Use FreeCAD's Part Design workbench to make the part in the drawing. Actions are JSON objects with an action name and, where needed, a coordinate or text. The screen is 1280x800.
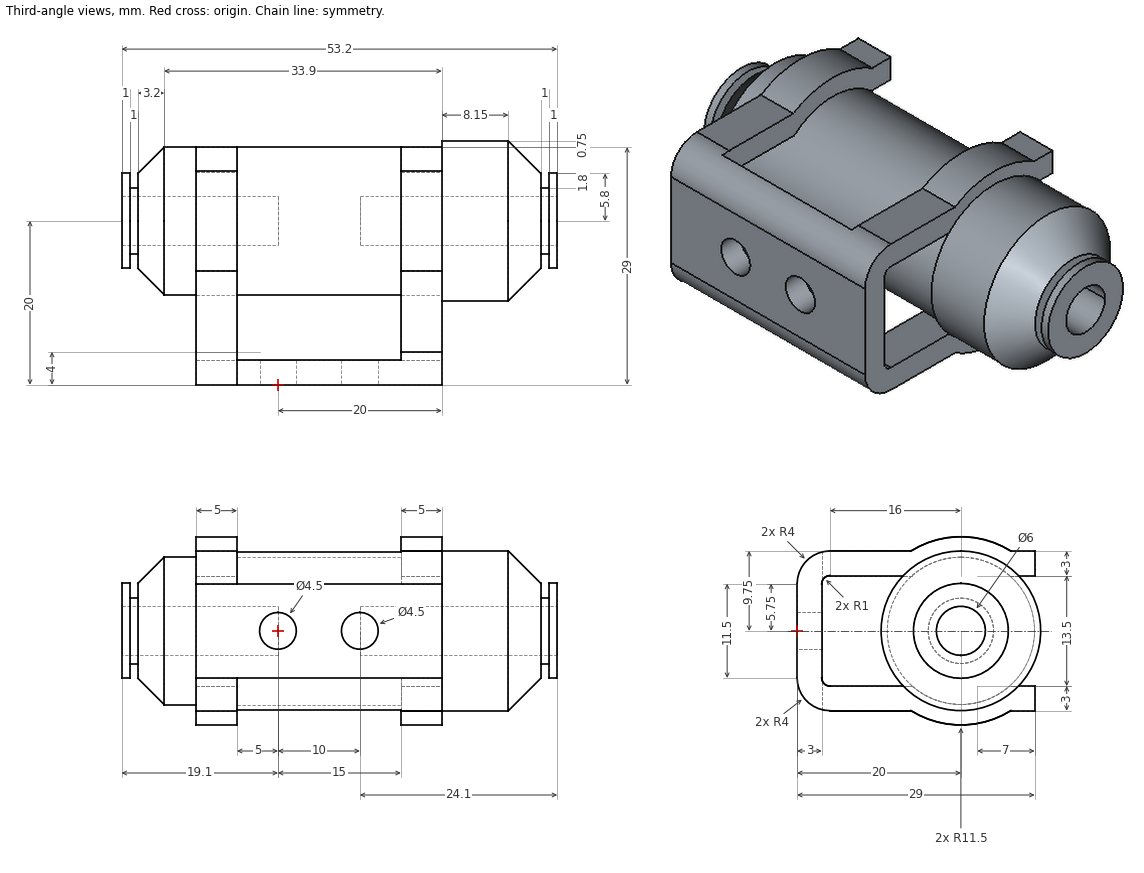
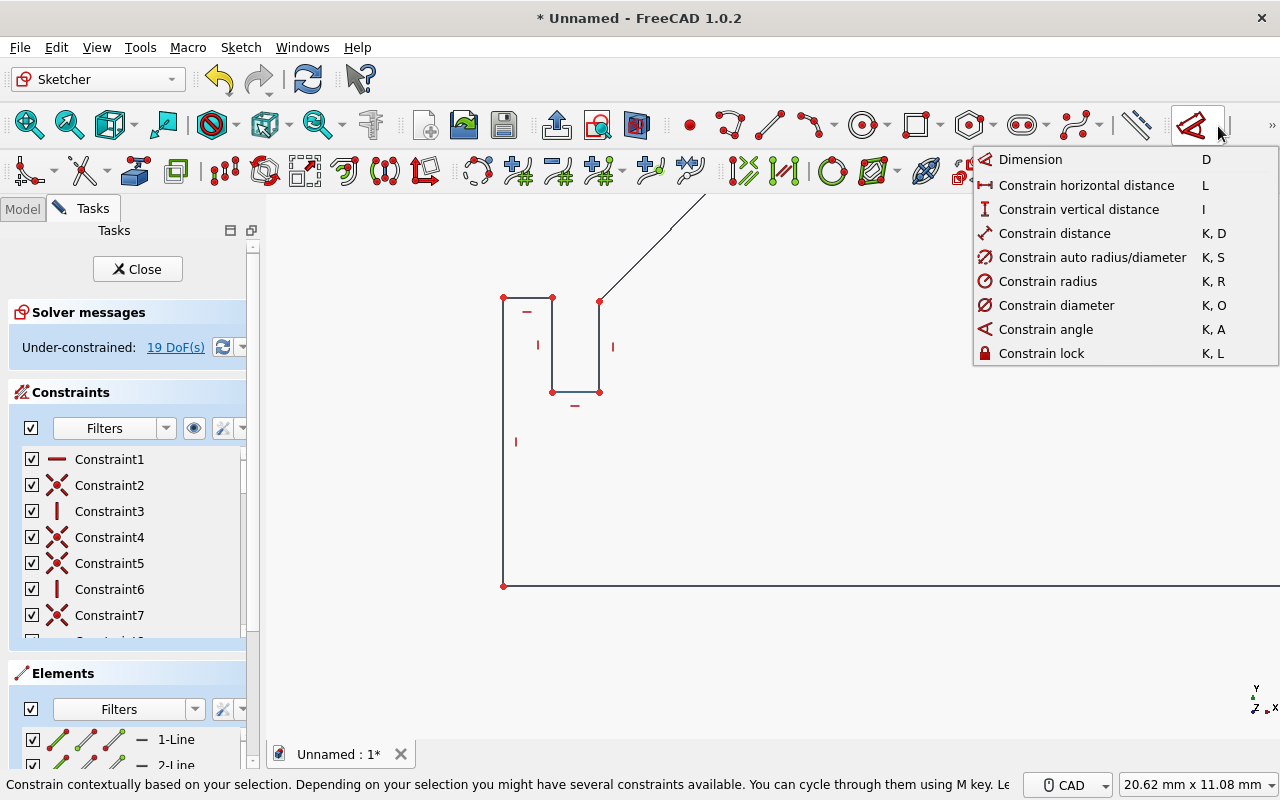
{"action": "left_click", "coordinate": [1126, 185]}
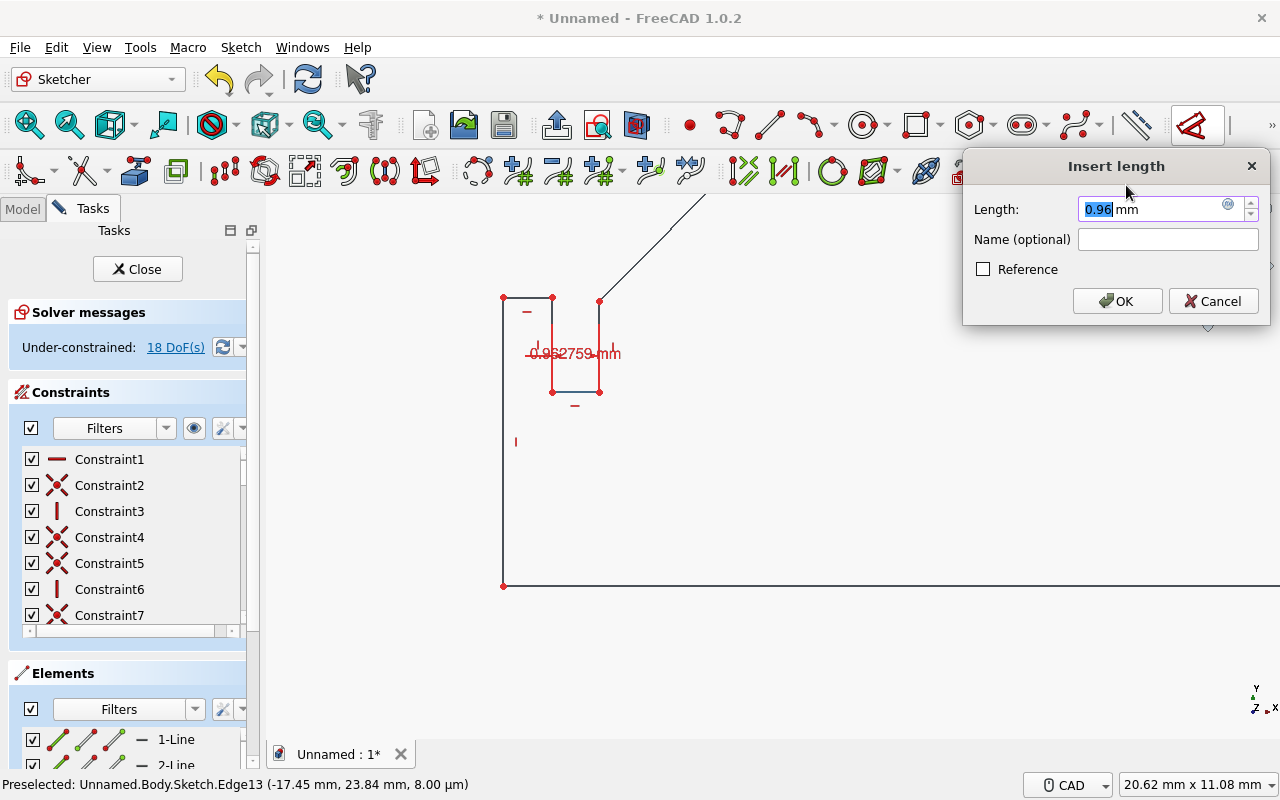
{"action": "type", "text": "1"}
{"action": "key", "text": "Return"}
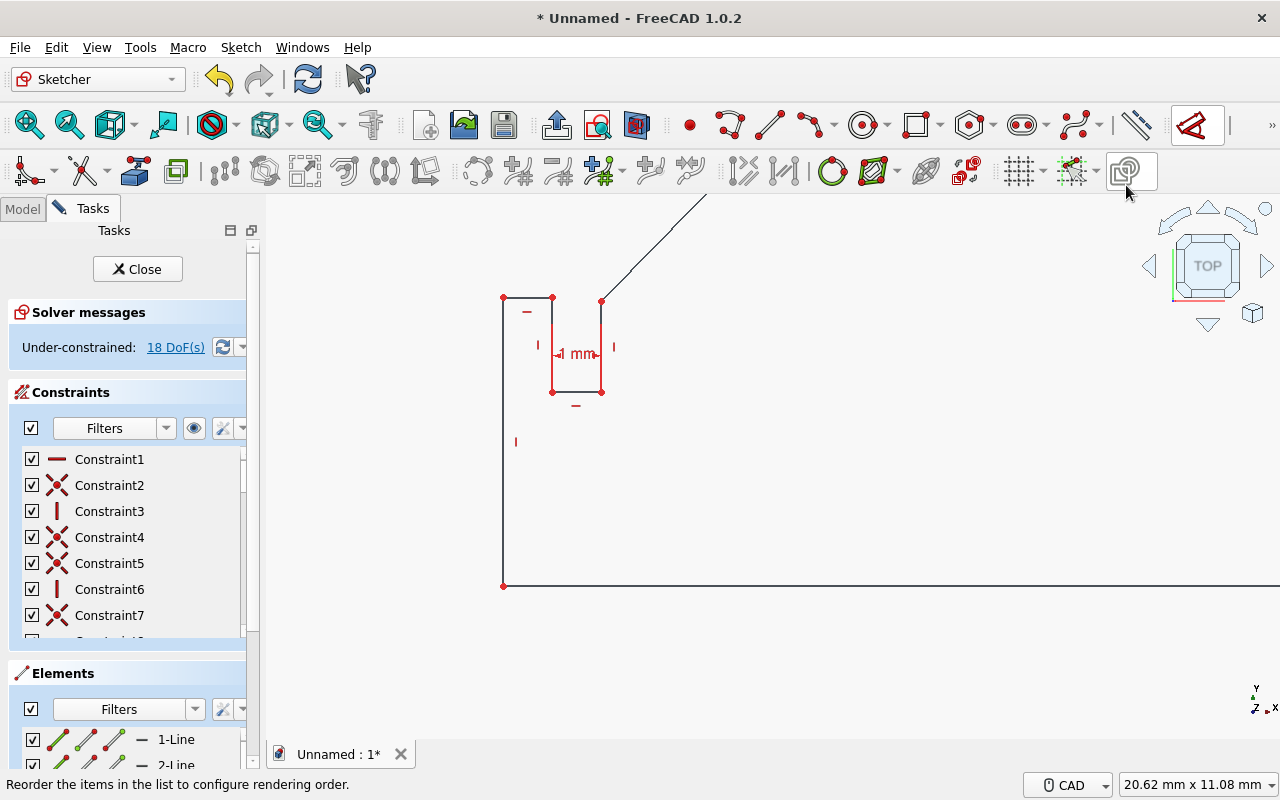
{"action": "left_click", "coordinate": [537, 298]}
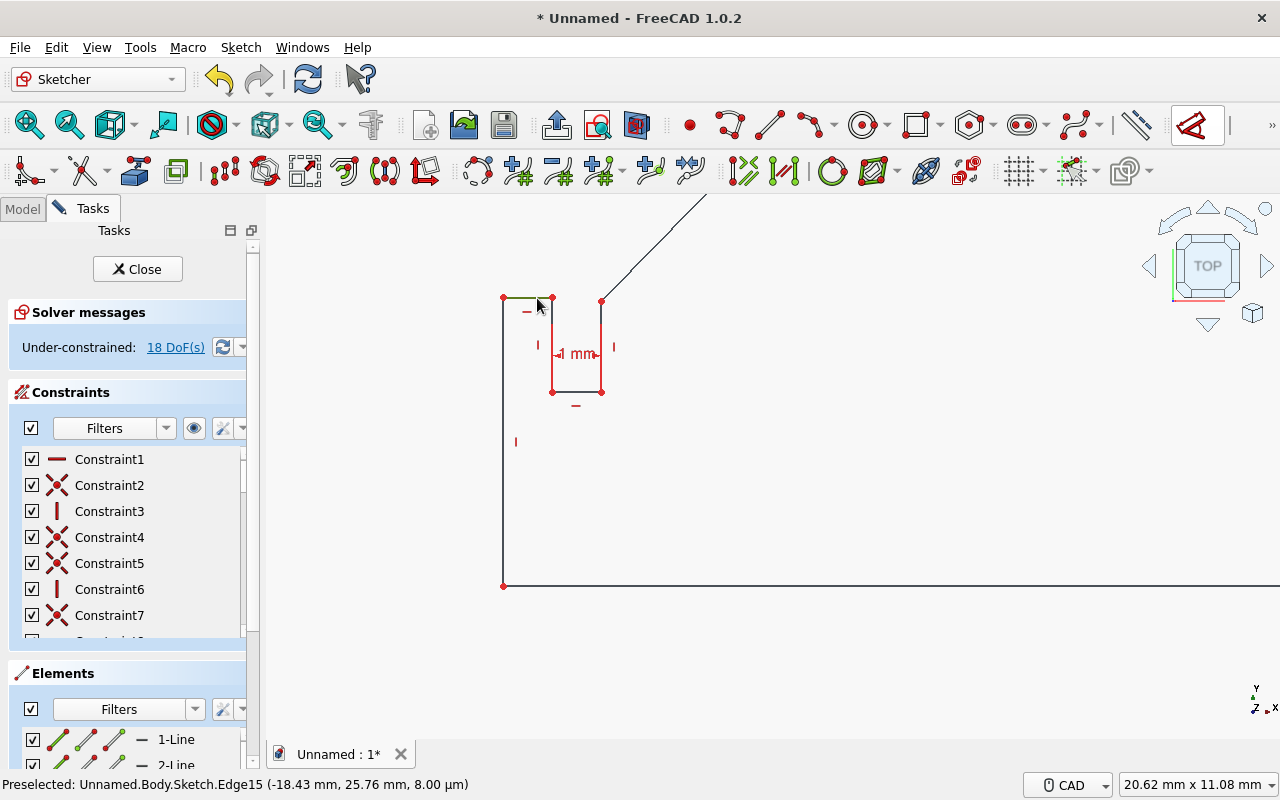
{"action": "key", "text": "l"}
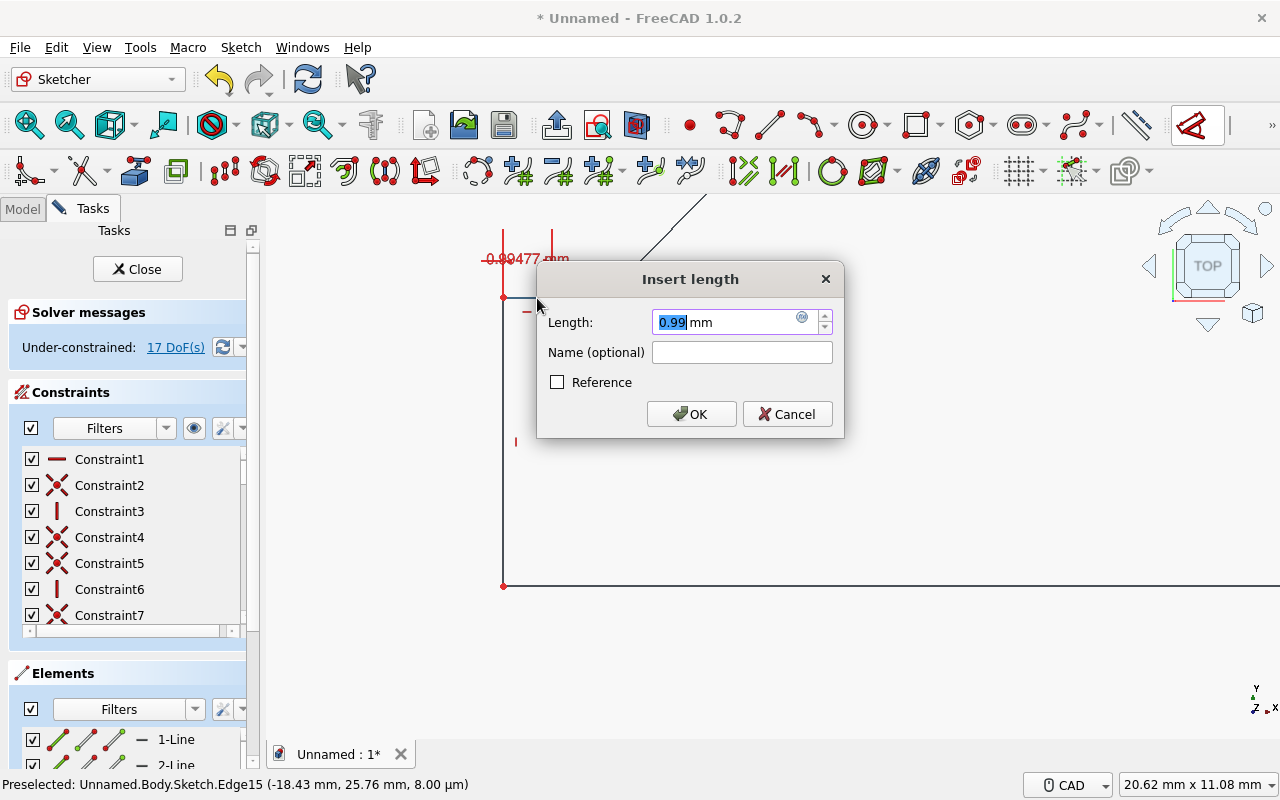
{"action": "type", "text": "1"}
{"action": "key", "text": "Return"}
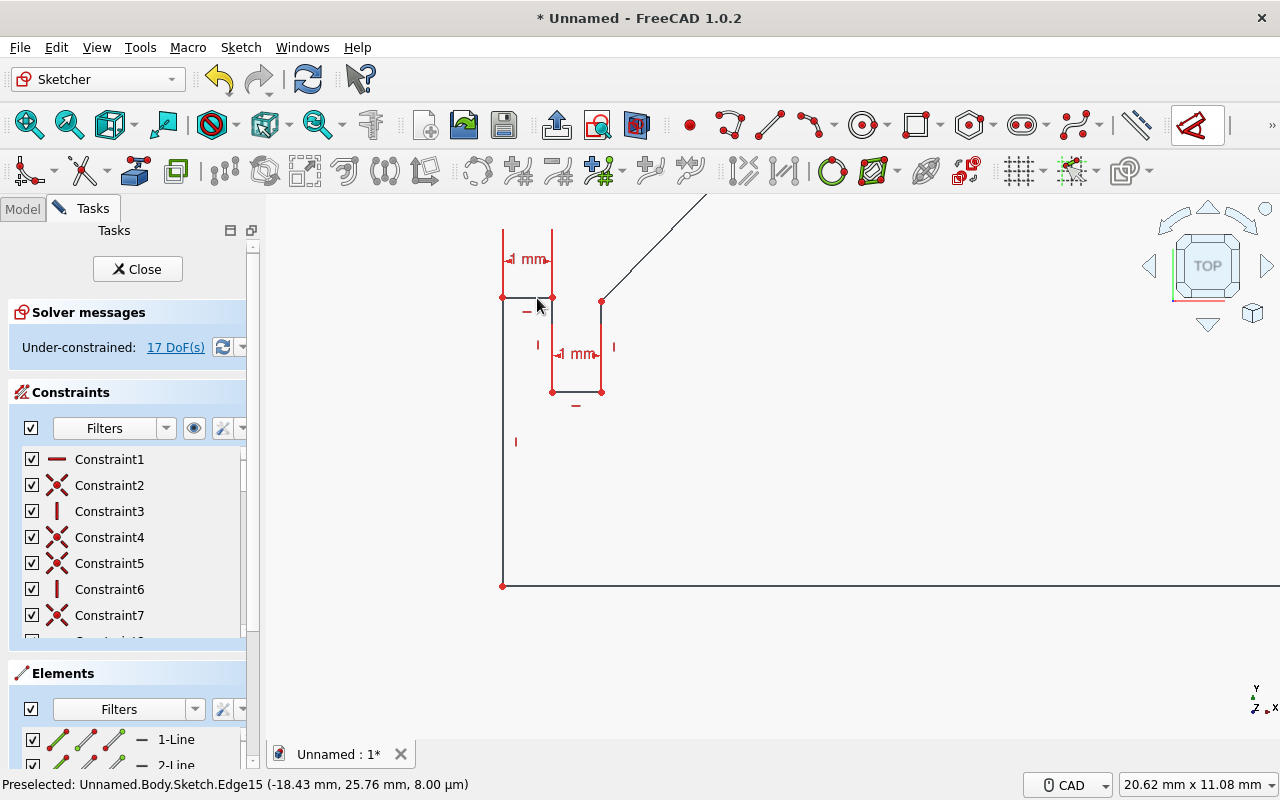
{"action": "scroll", "coordinate": [589, 394], "scroll_direction": "down", "scroll_amount": 9}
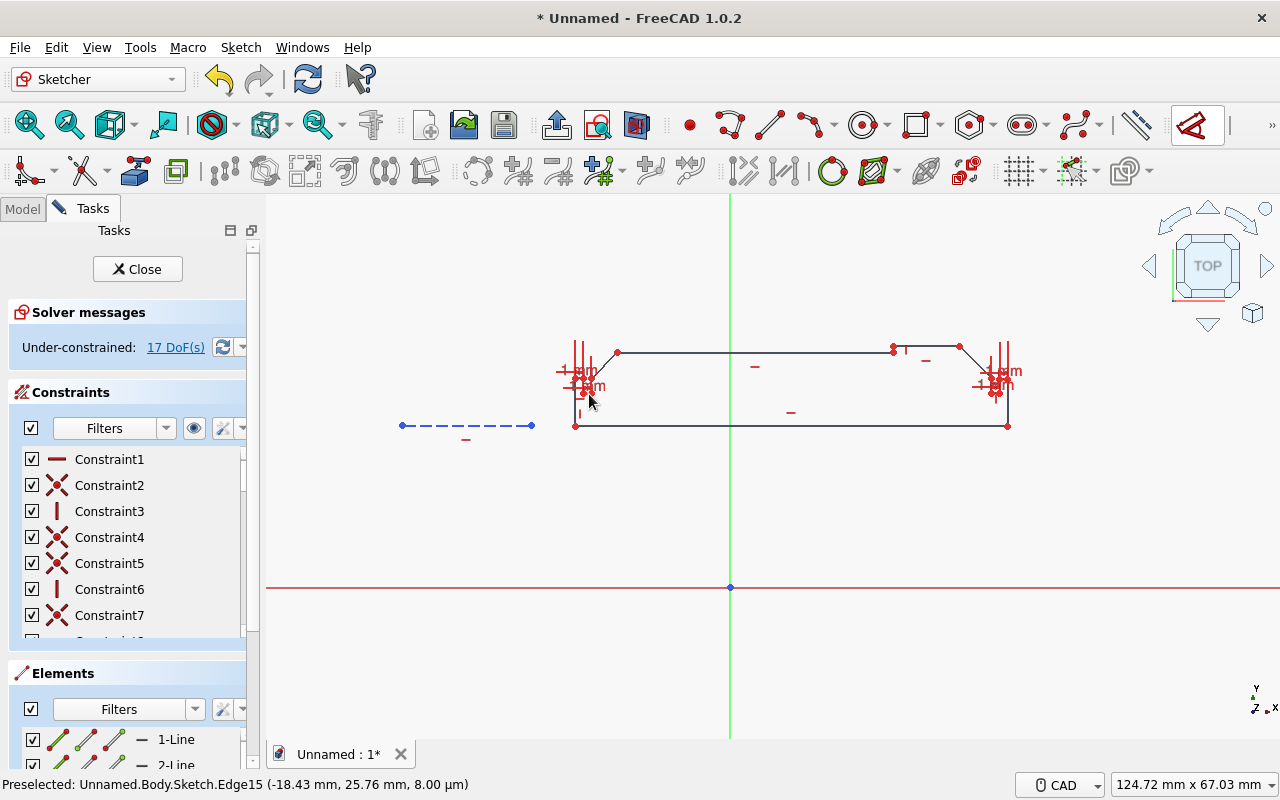
{"action": "left_click", "coordinate": [1008, 412]}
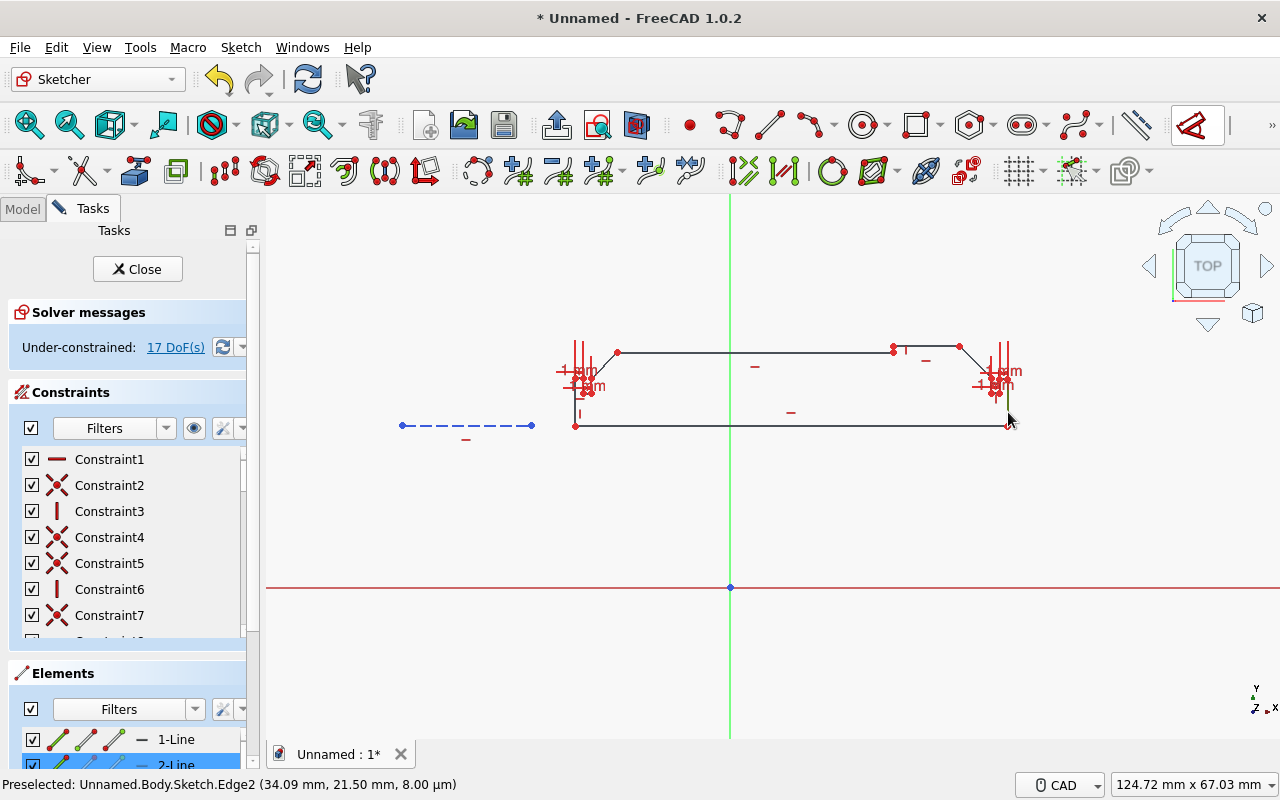
{"action": "left_click", "coordinate": [1218, 126]}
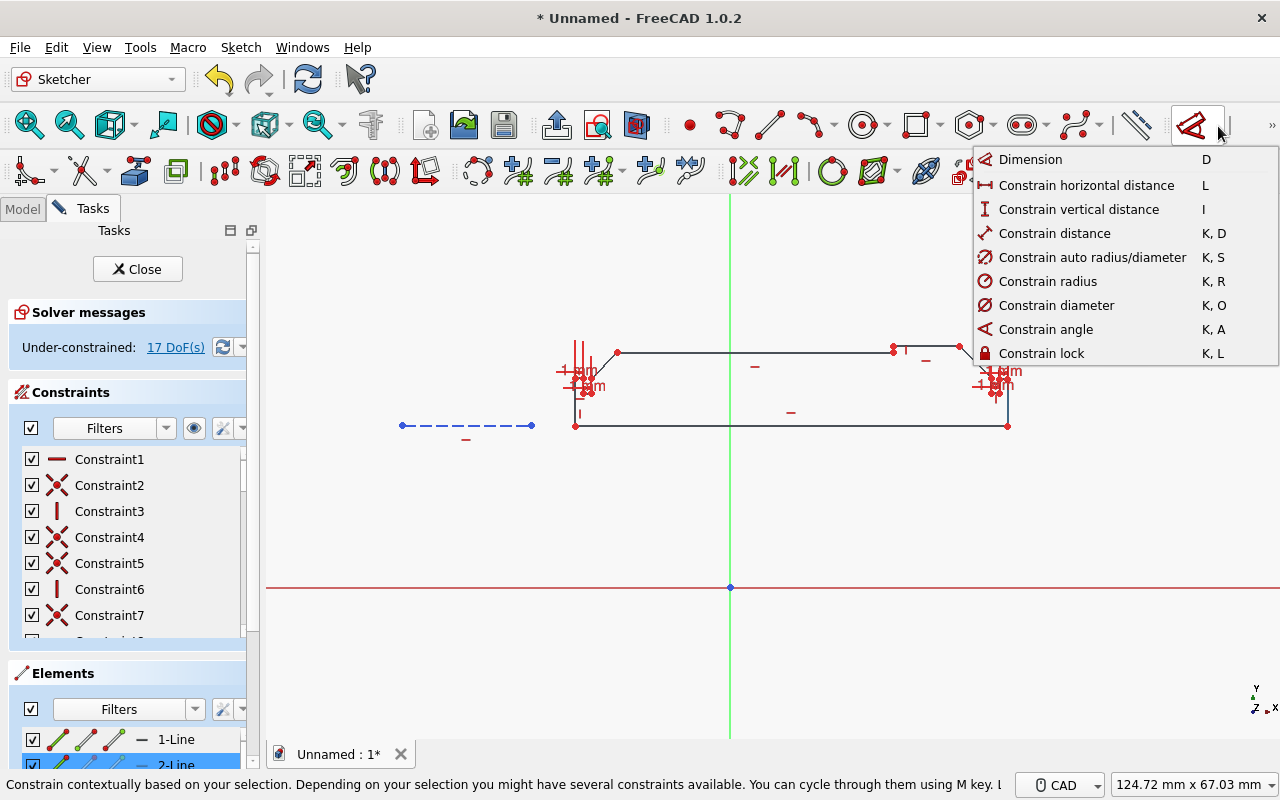
{"action": "left_click", "coordinate": [1126, 209]}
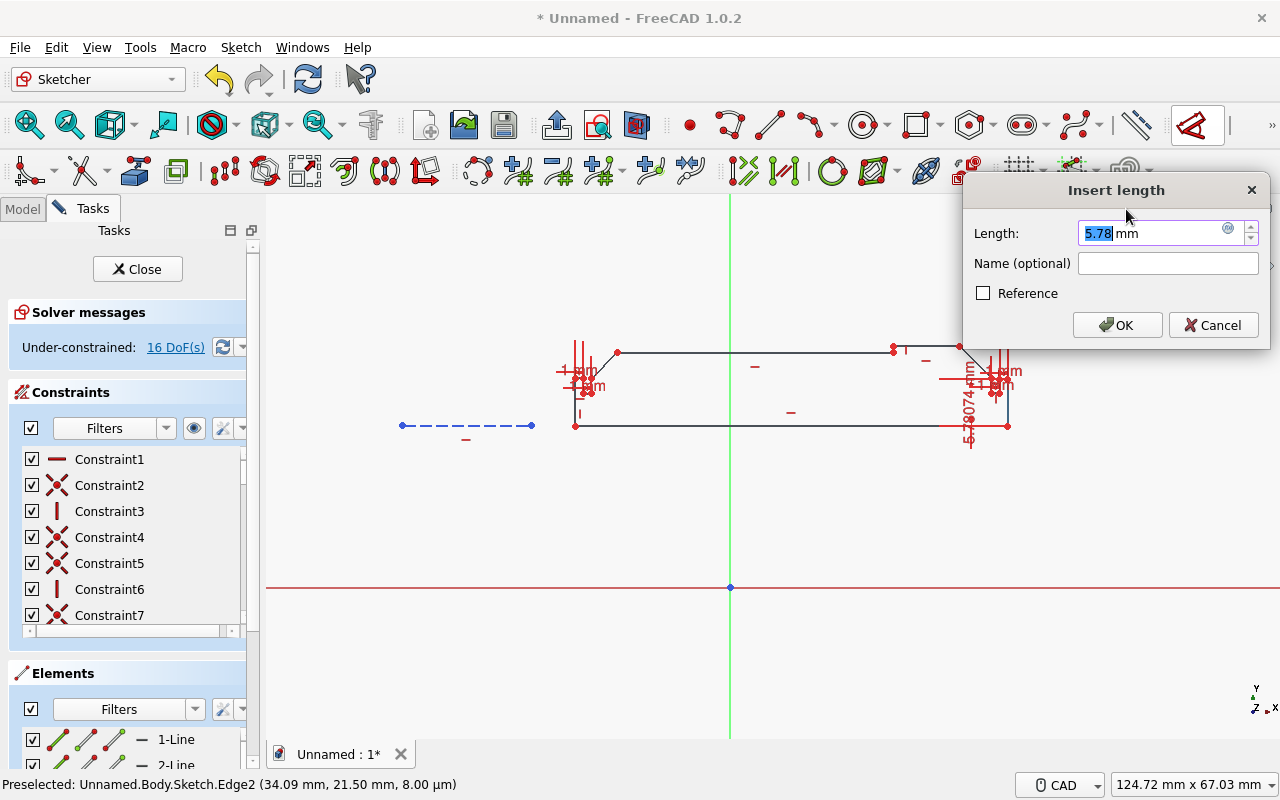
{"action": "type", "text": "5.8"}
{"action": "key", "text": "Return"}